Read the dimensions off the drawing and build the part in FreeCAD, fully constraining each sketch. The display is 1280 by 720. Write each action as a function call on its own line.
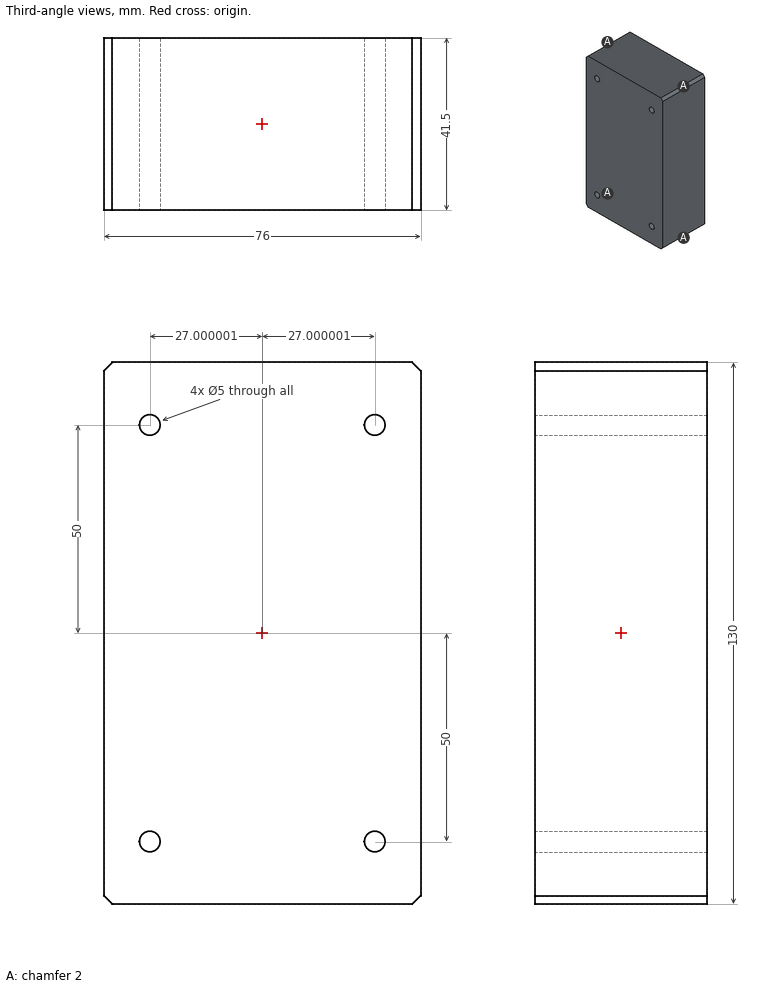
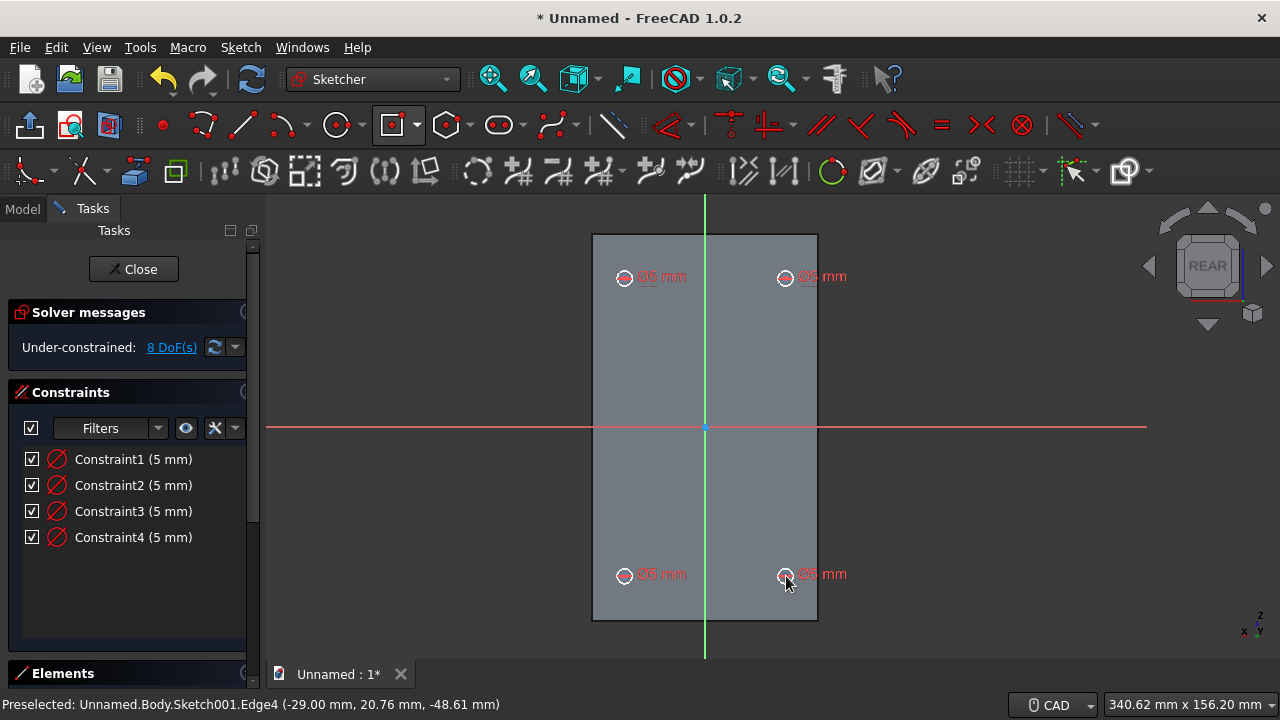
click(786, 279)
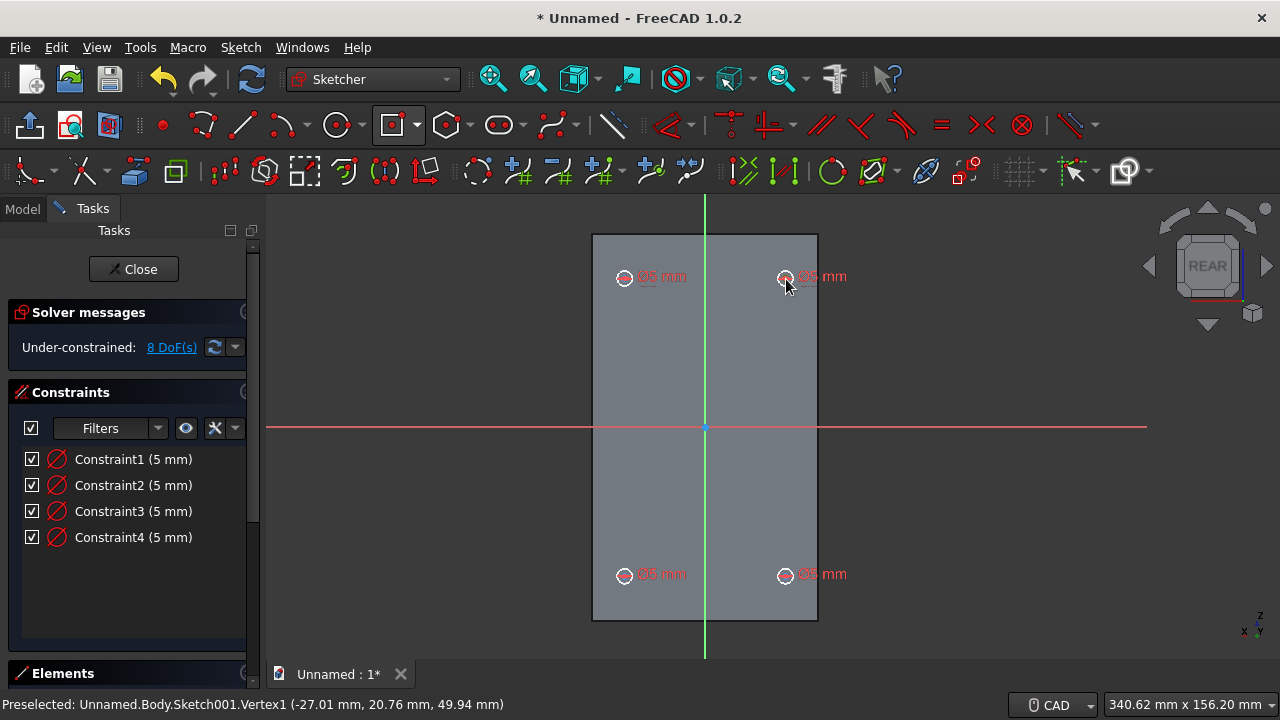
click(625, 279)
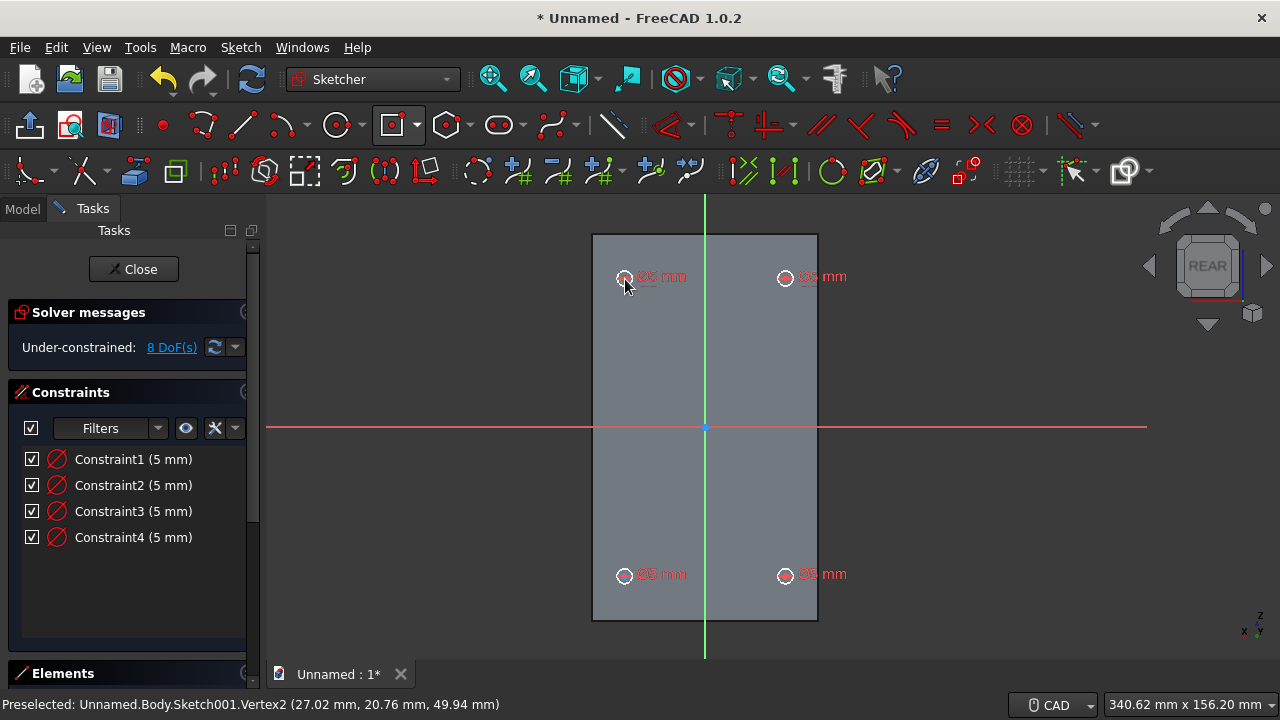
click(796, 126)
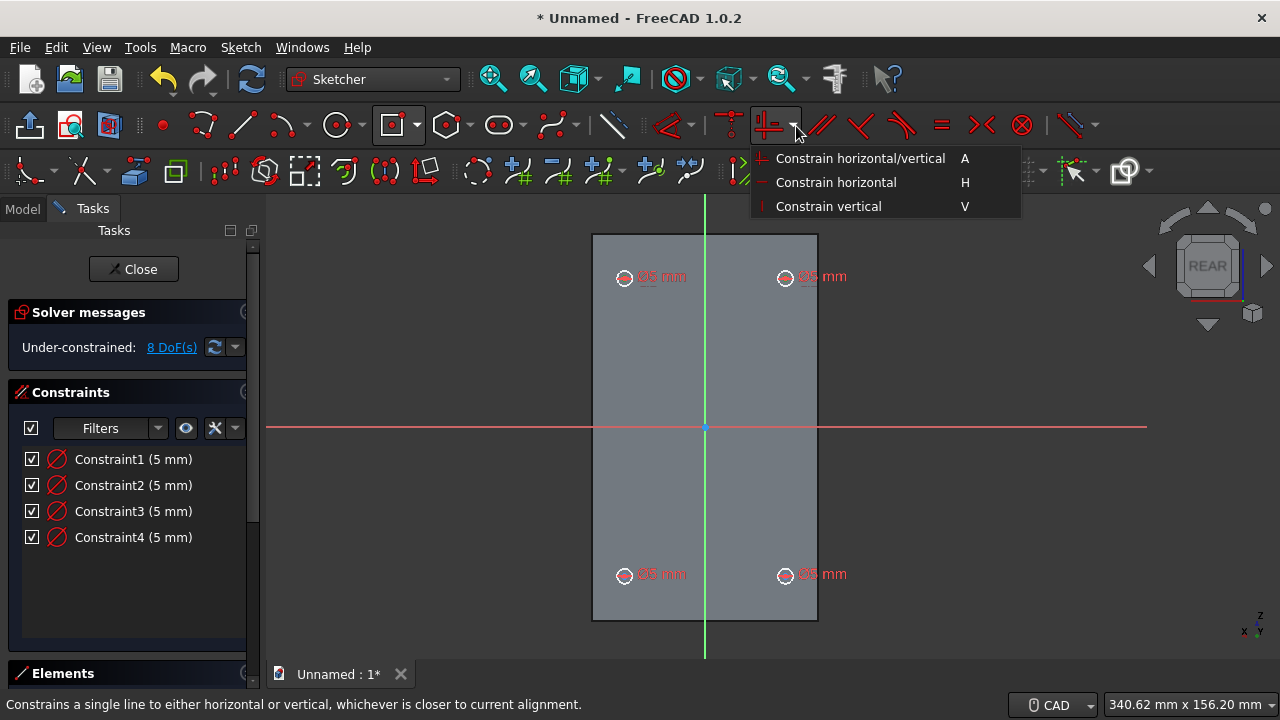
click(886, 182)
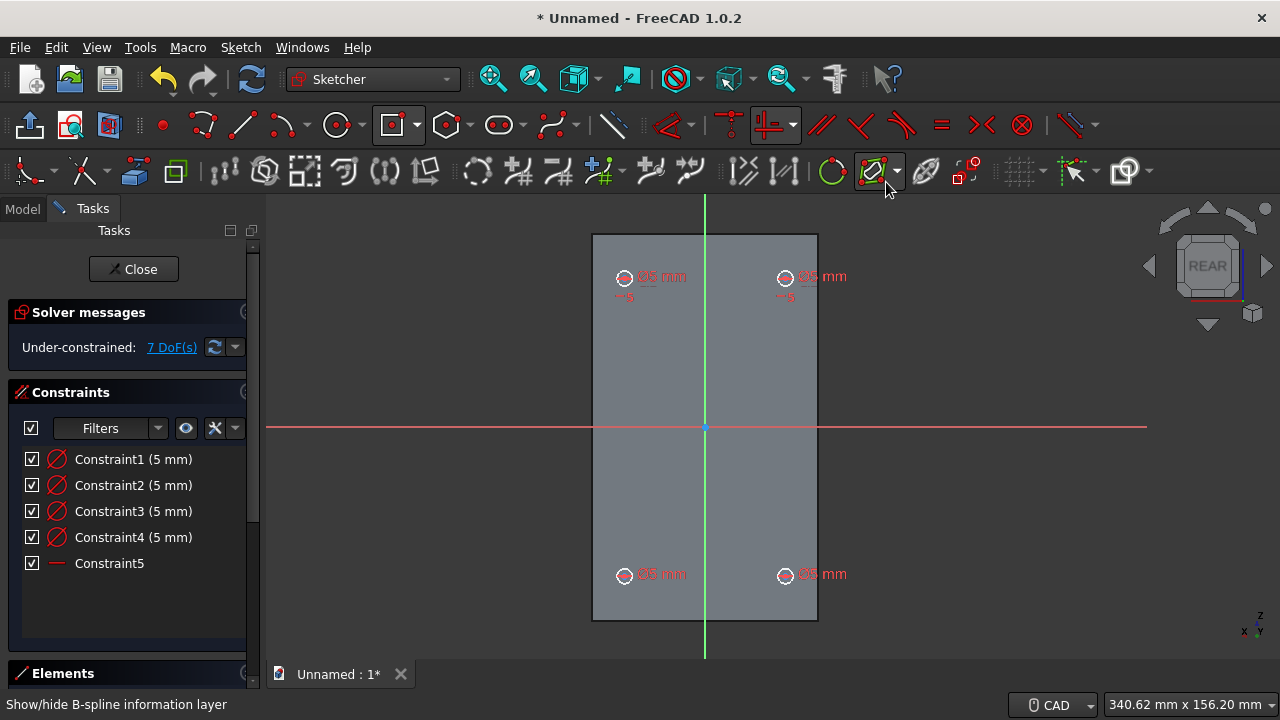
click(625, 279)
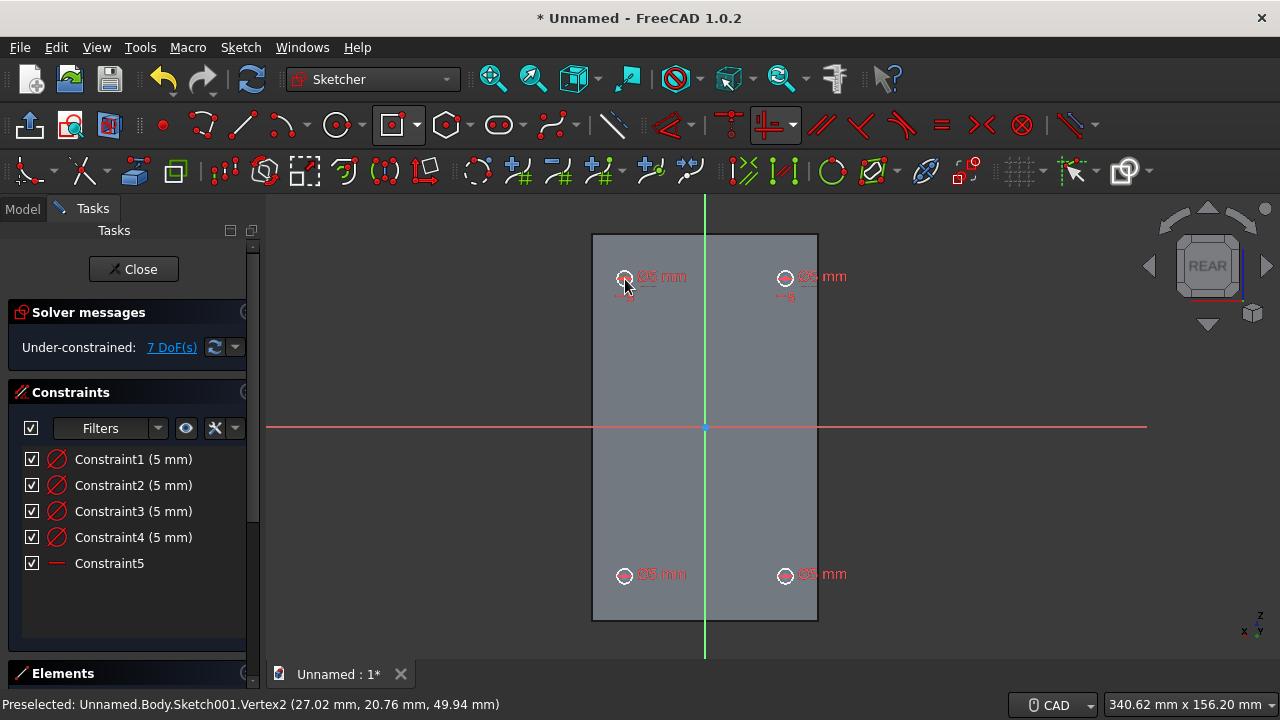
click(625, 576)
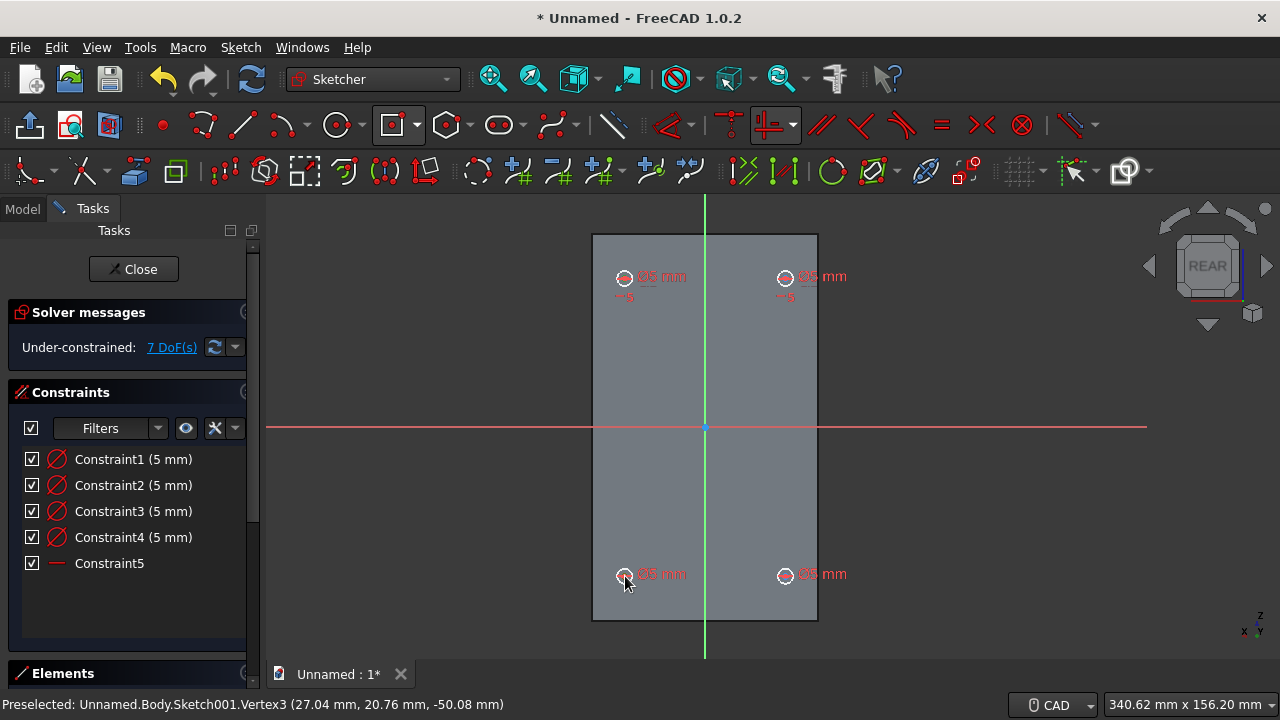
click(796, 126)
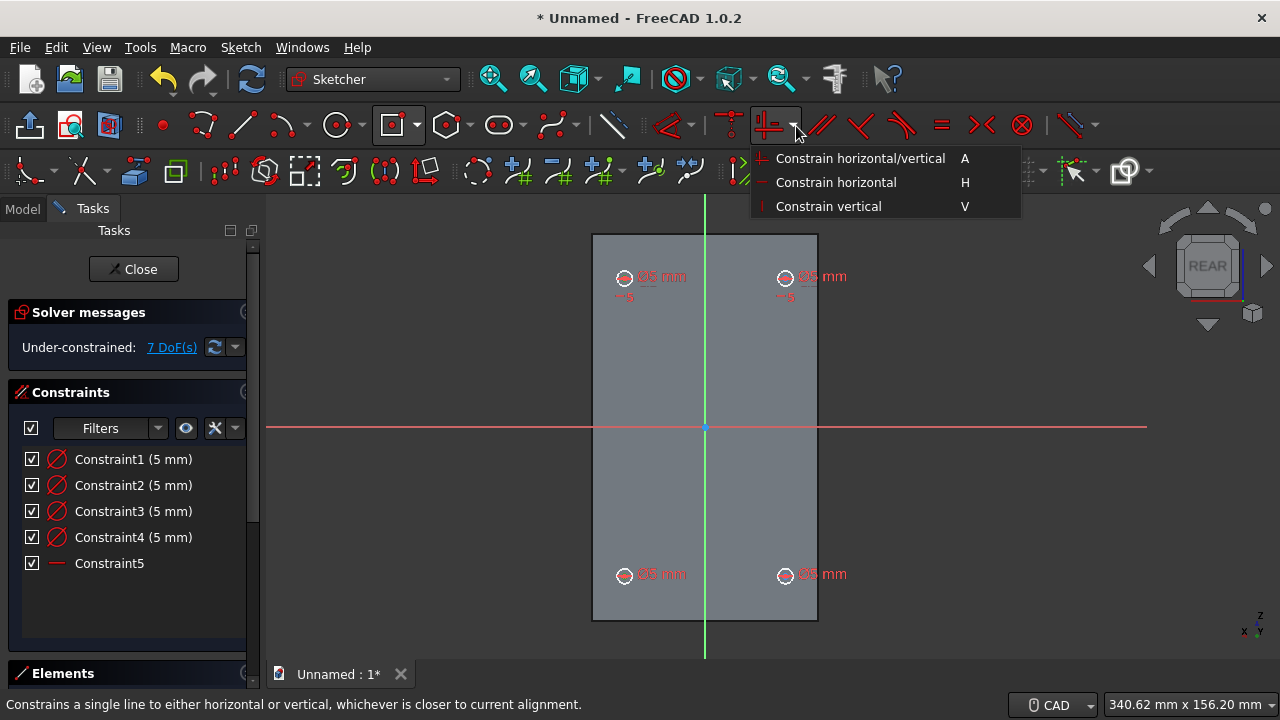
click(886, 206)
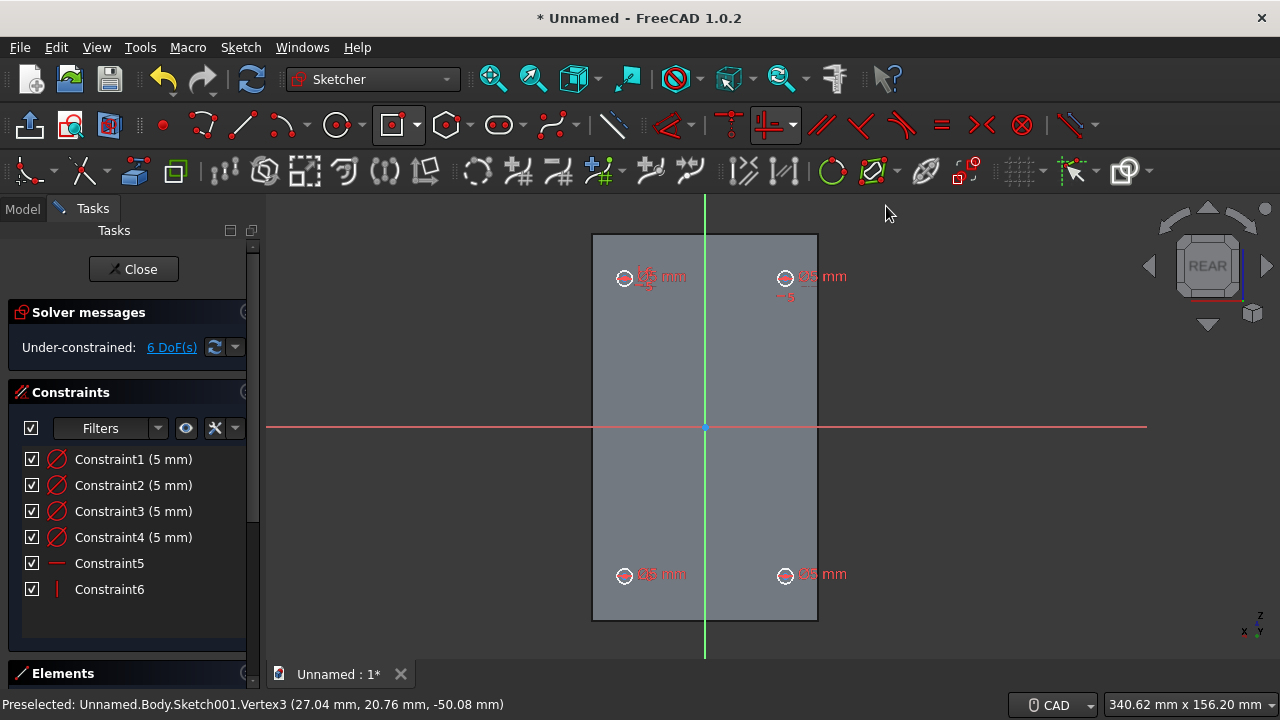
click(786, 279)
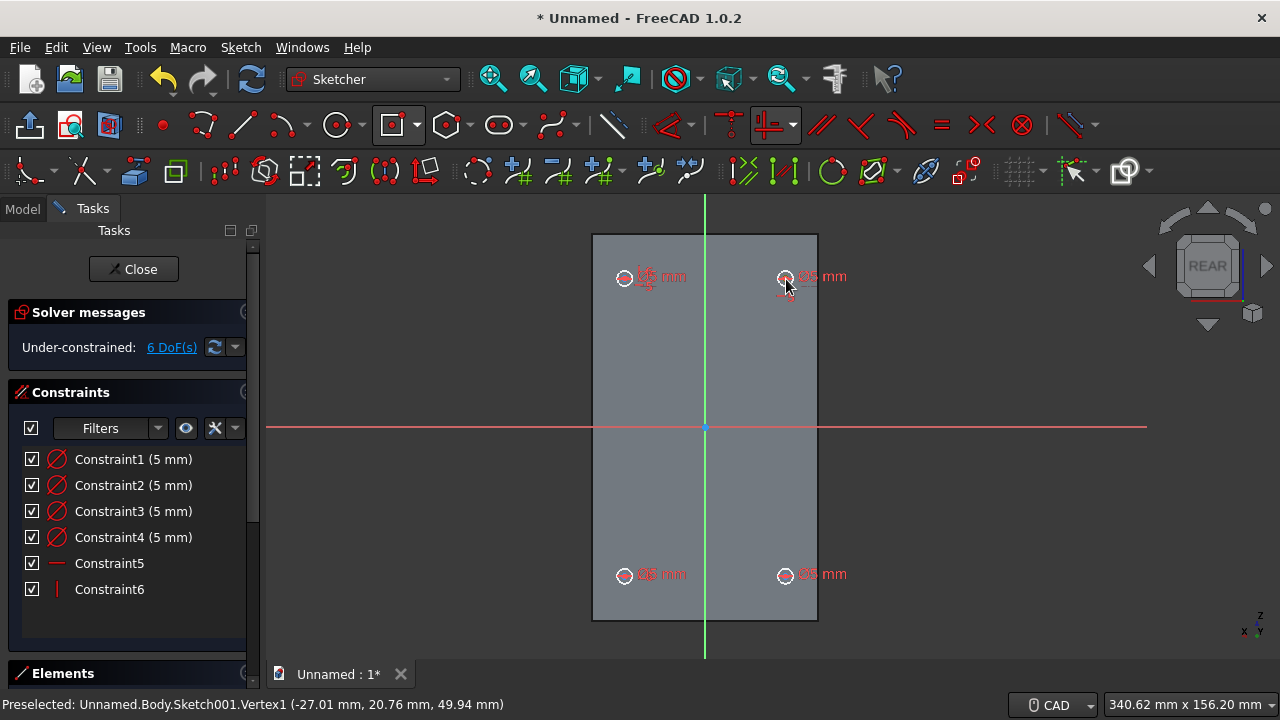
click(785, 576)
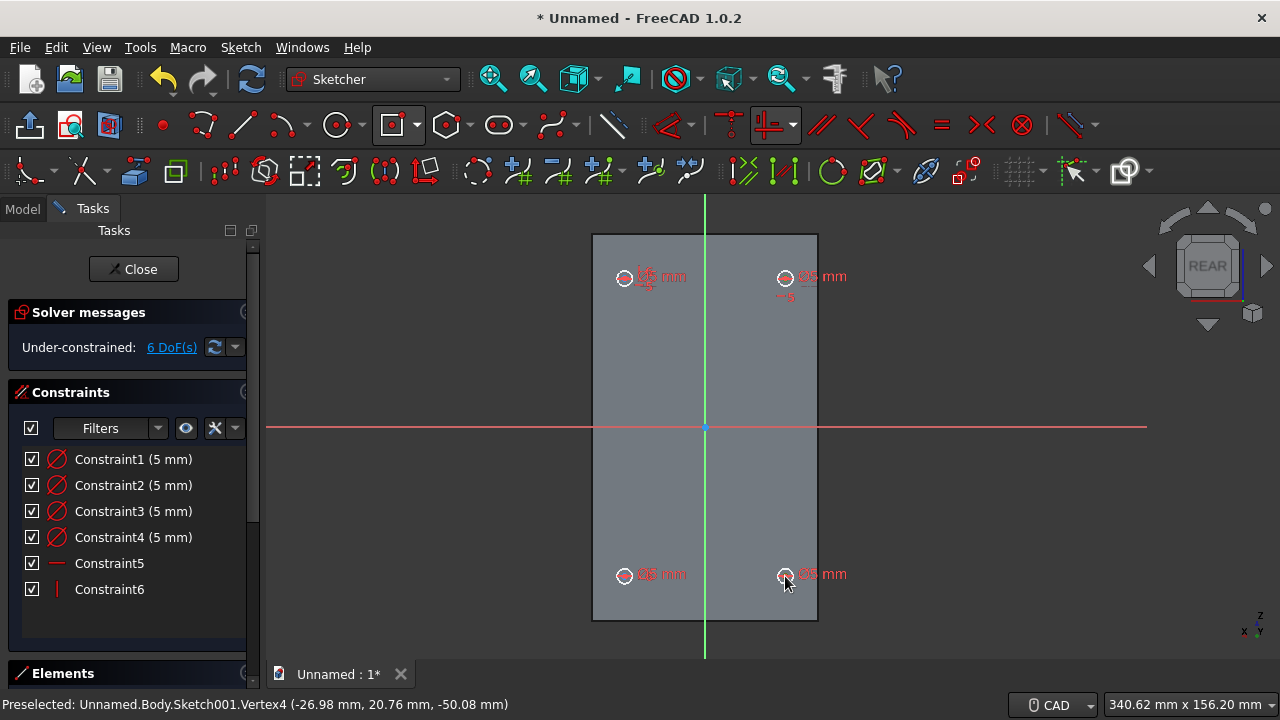
click(796, 126)